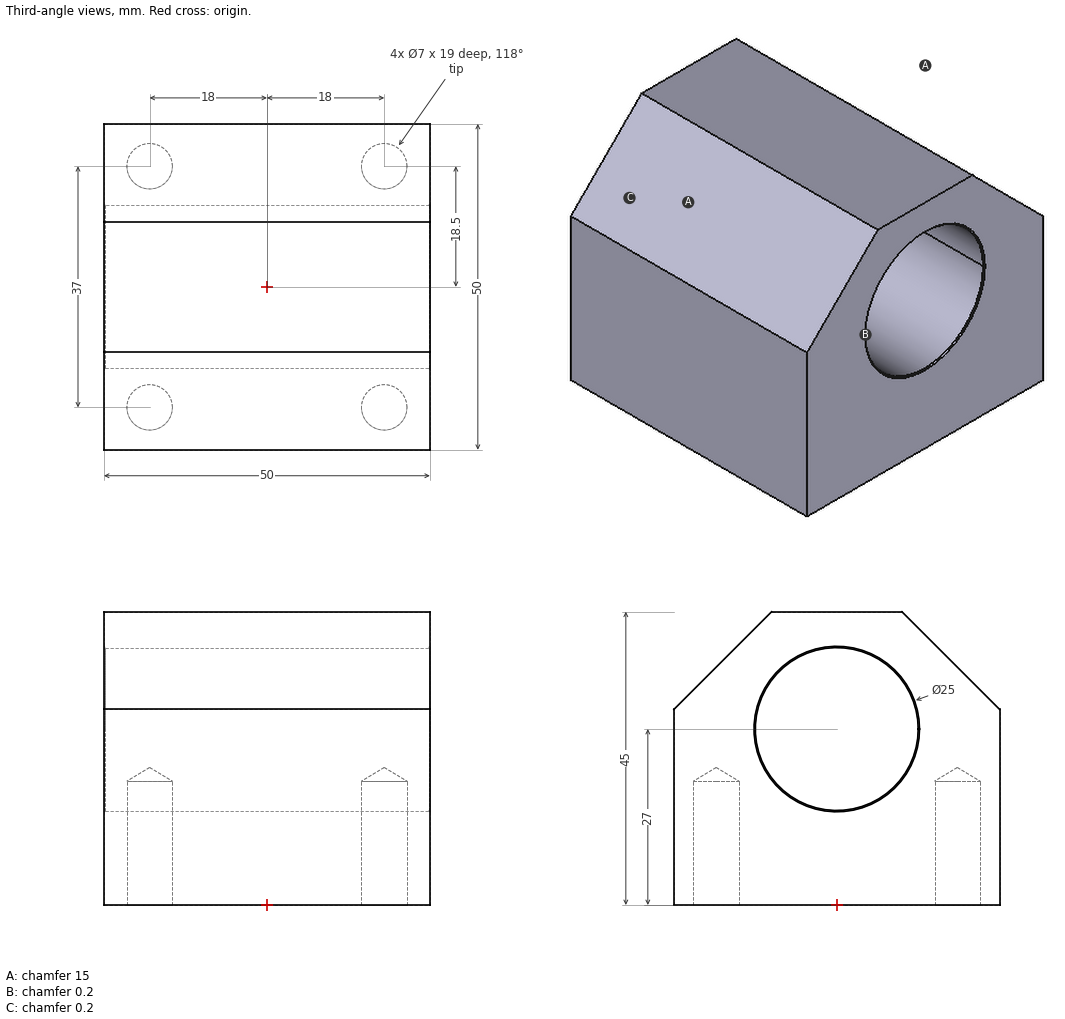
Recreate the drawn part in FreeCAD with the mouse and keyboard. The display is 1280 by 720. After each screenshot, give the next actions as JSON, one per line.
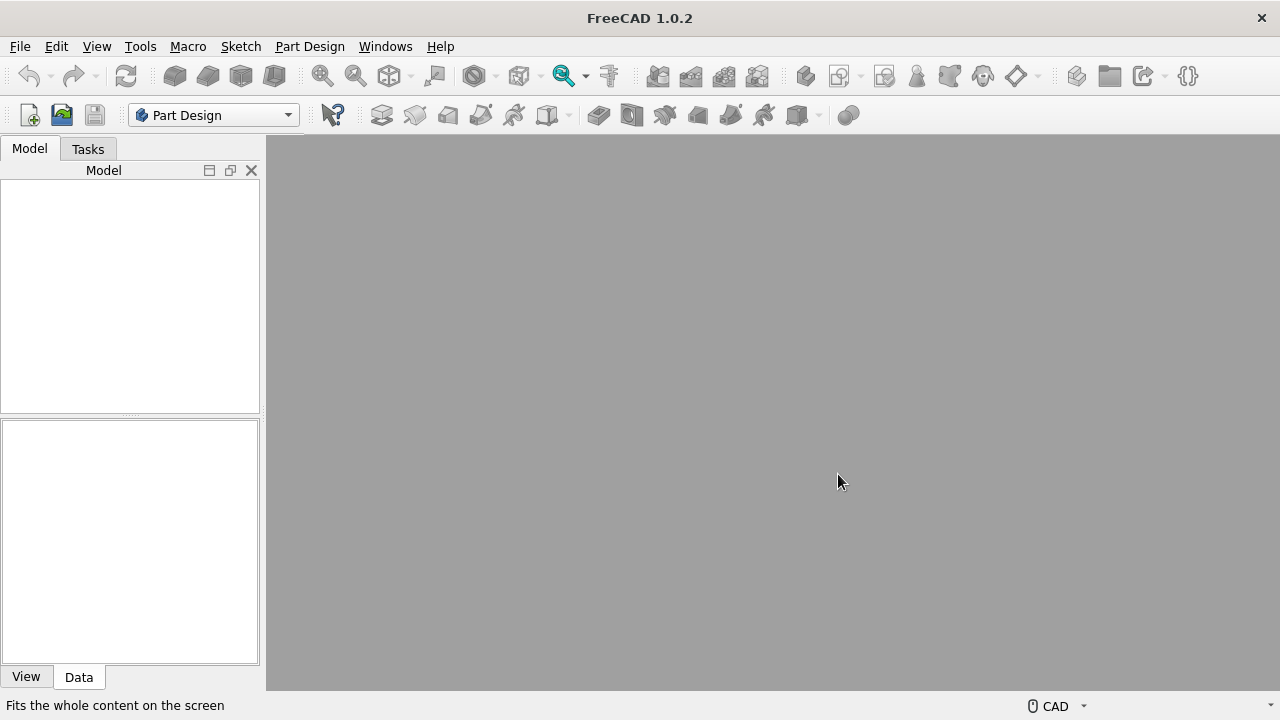
{"action": "left_click", "coordinate": [29, 116]}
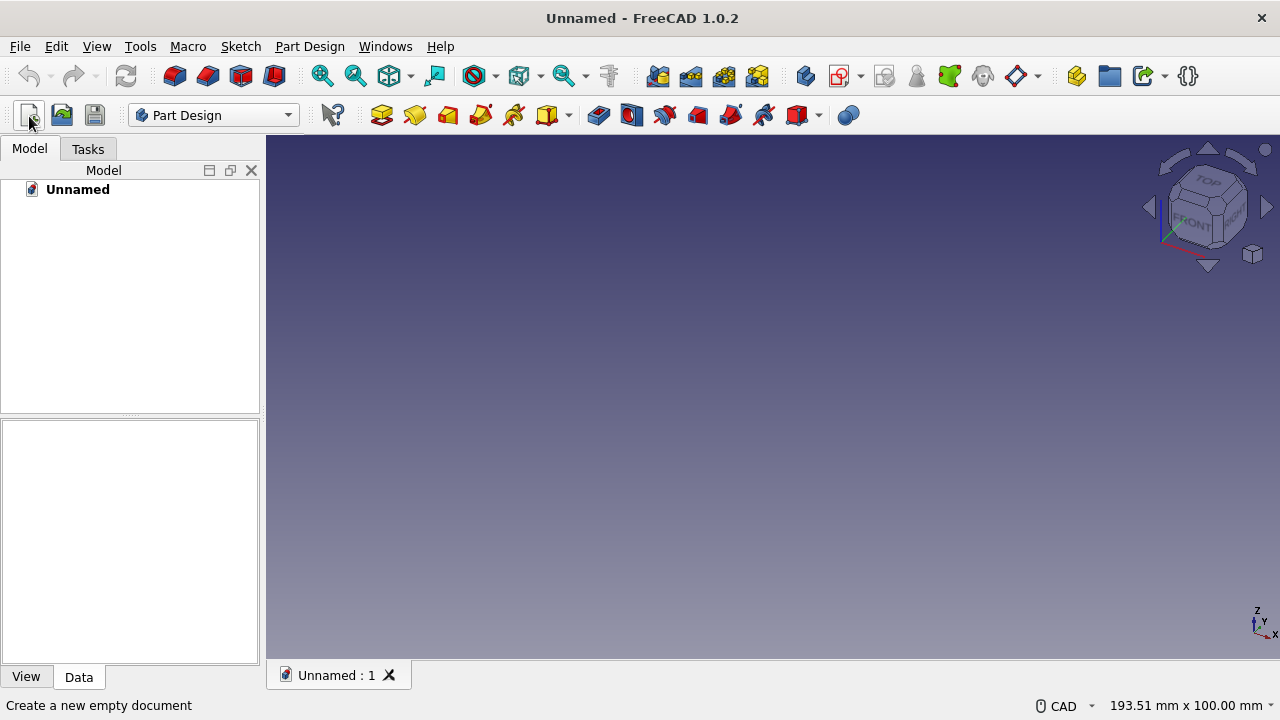
{"action": "left_click", "coordinate": [838, 76]}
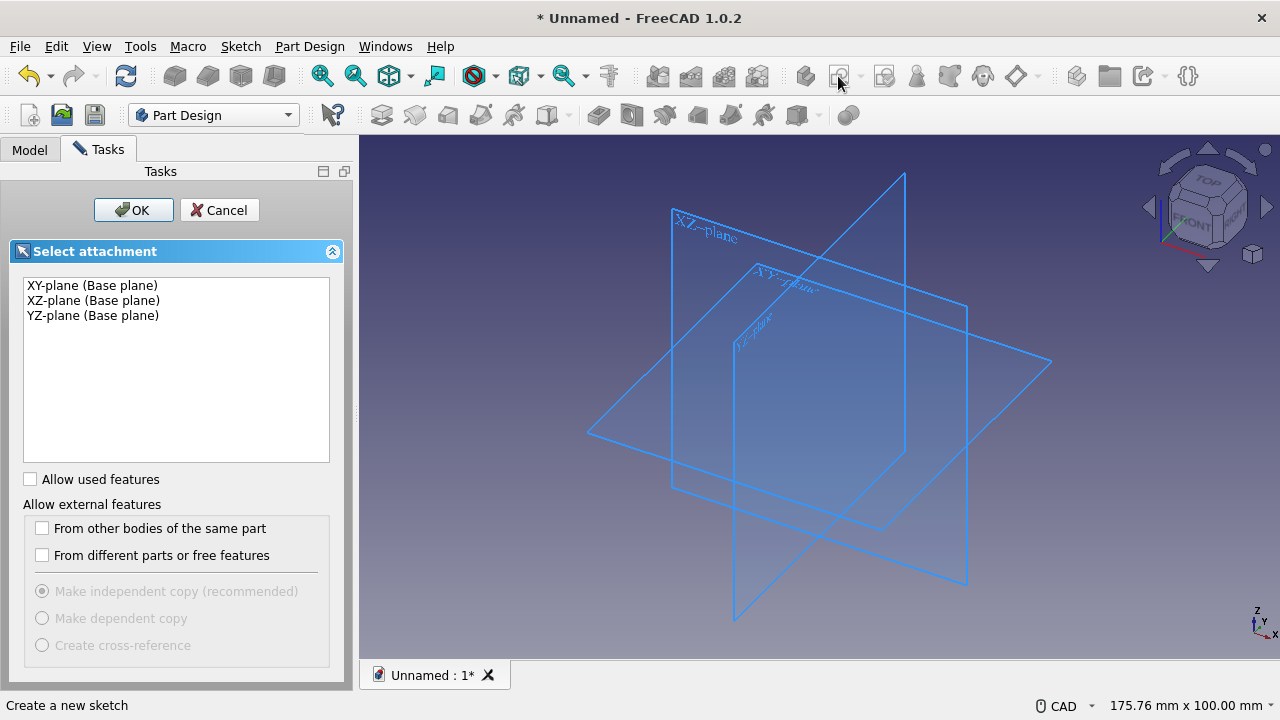
{"action": "left_click", "coordinate": [84, 286]}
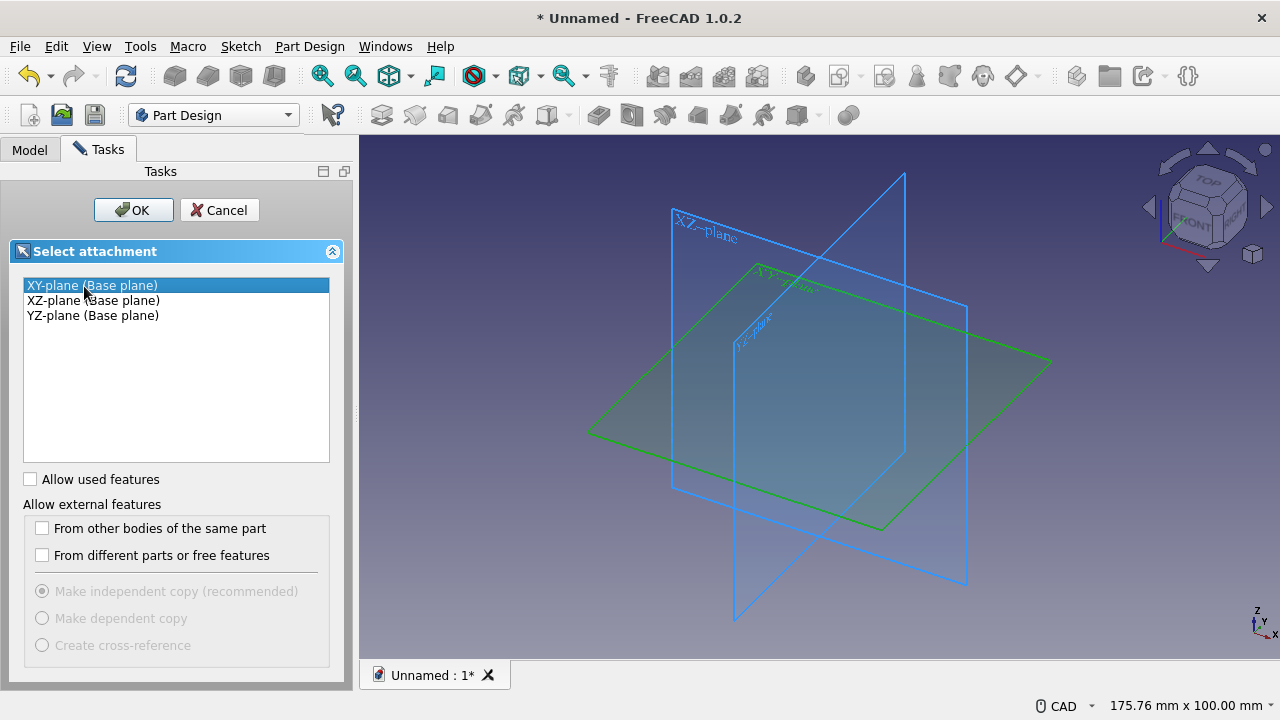
{"action": "left_click", "coordinate": [134, 210]}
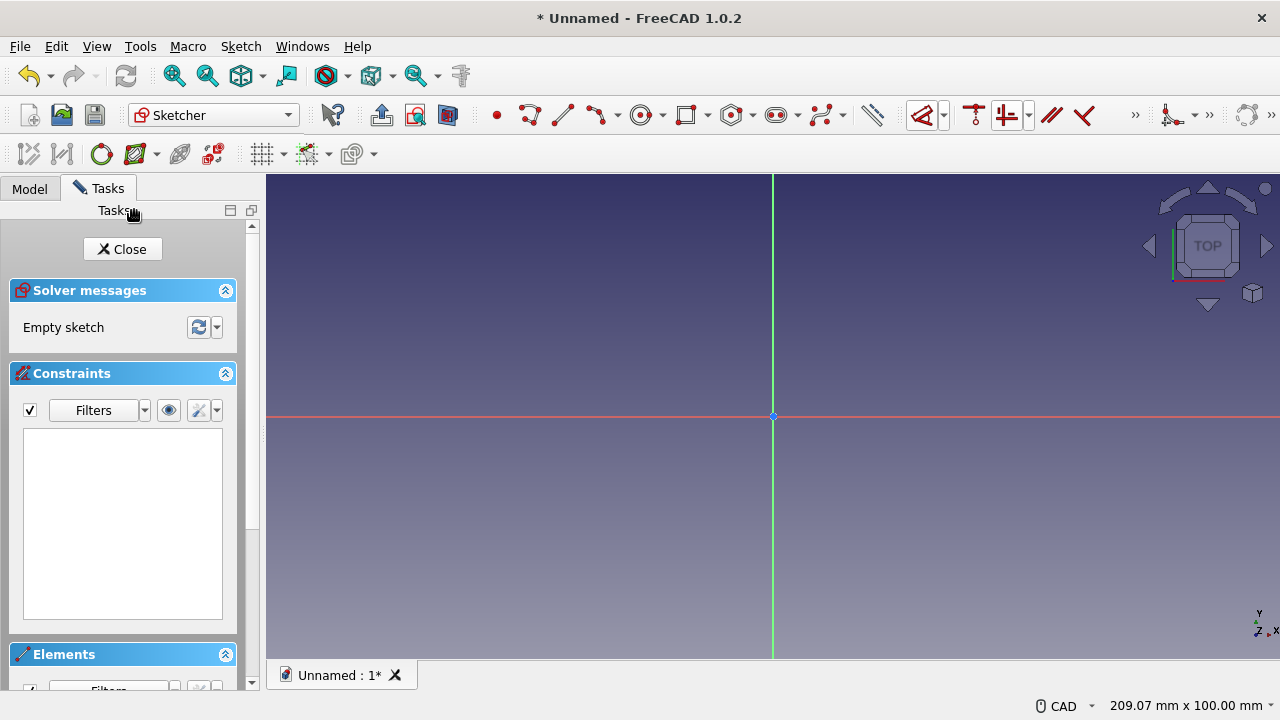
{"action": "left_click", "coordinate": [708, 116]}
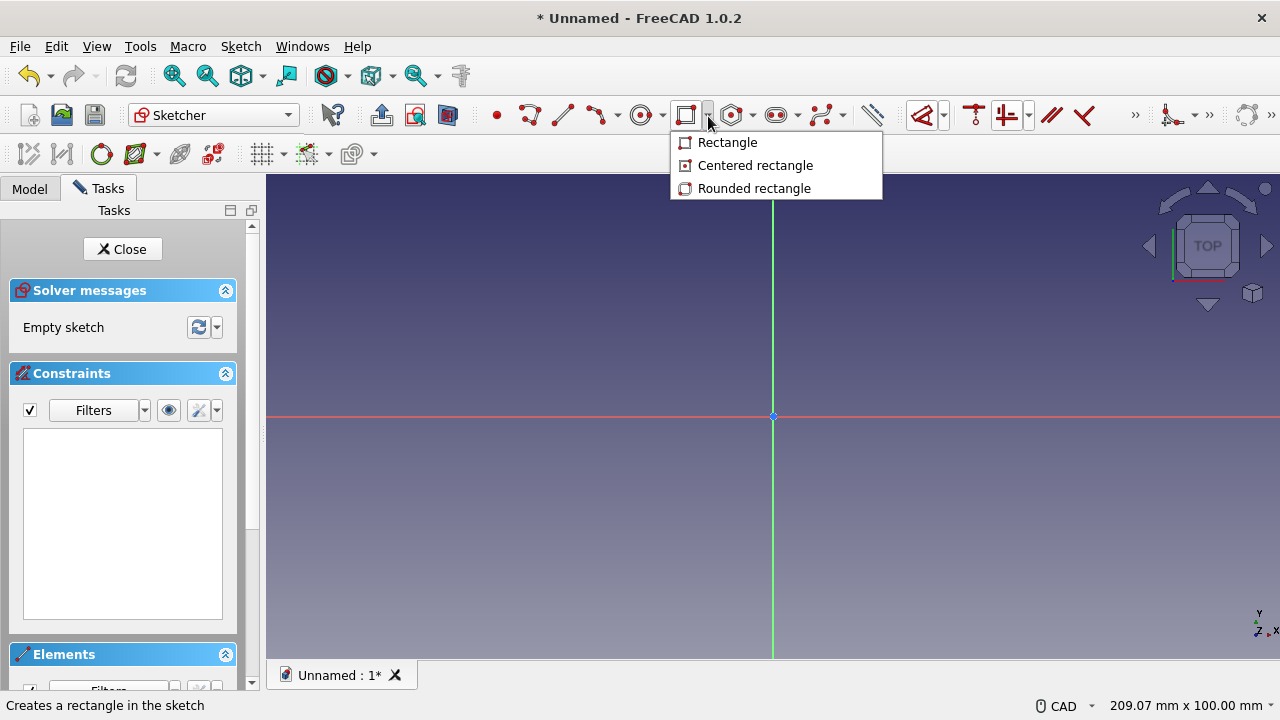
{"action": "left_click", "coordinate": [776, 166]}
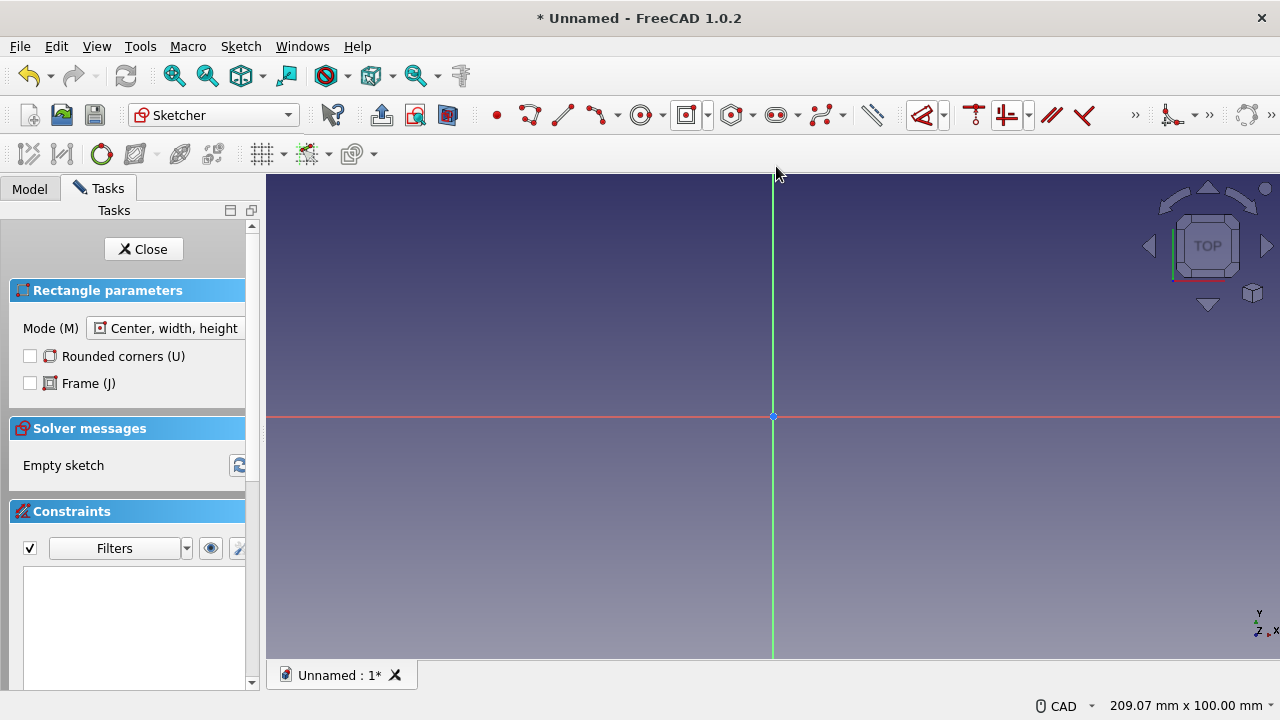
{"action": "left_click", "coordinate": [773, 416]}
{"action": "left_click", "coordinate": [894, 295]}
{"action": "key", "text": "Escape"}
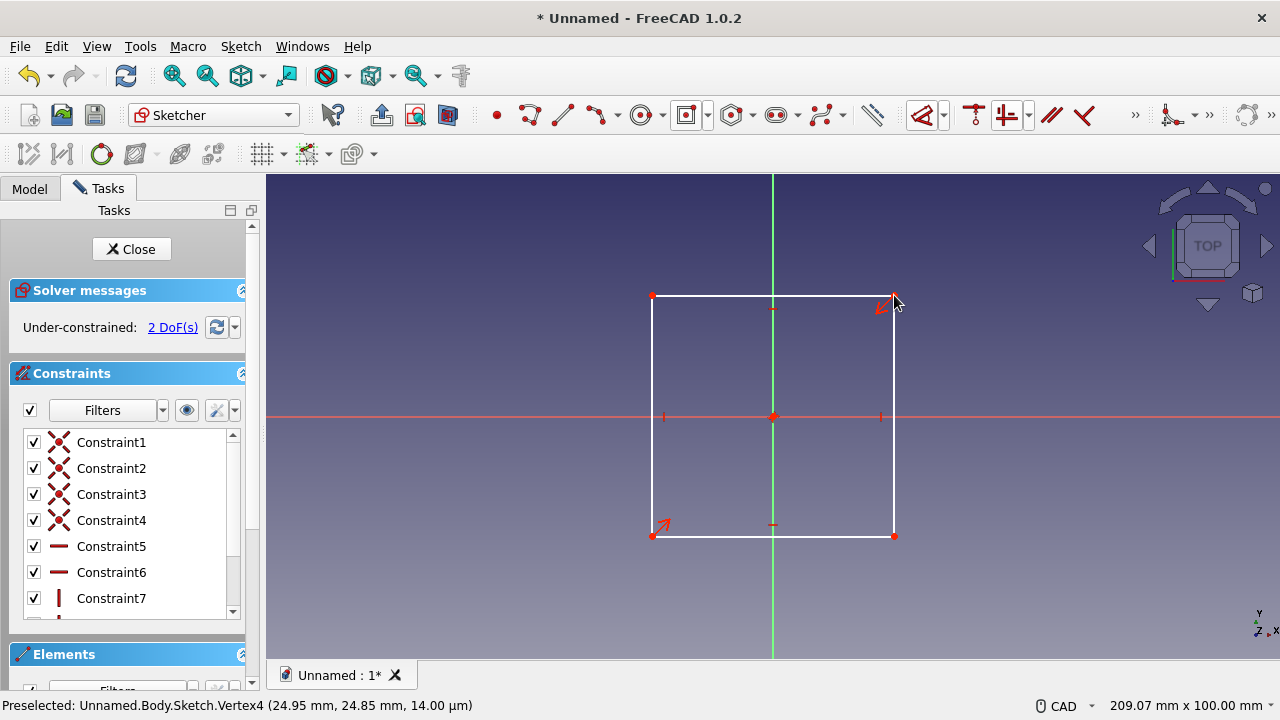
{"action": "left_click", "coordinate": [922, 116]}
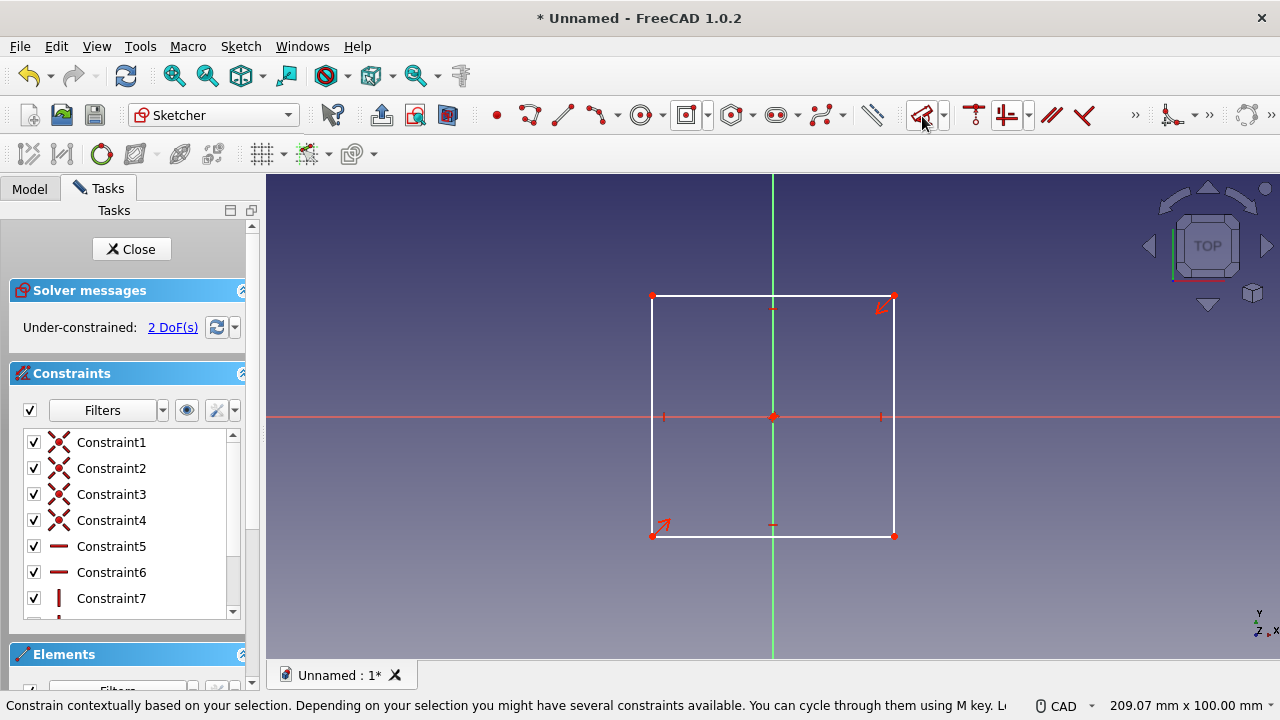
{"action": "left_click", "coordinate": [725, 537]}
{"action": "left_click", "coordinate": [717, 571]}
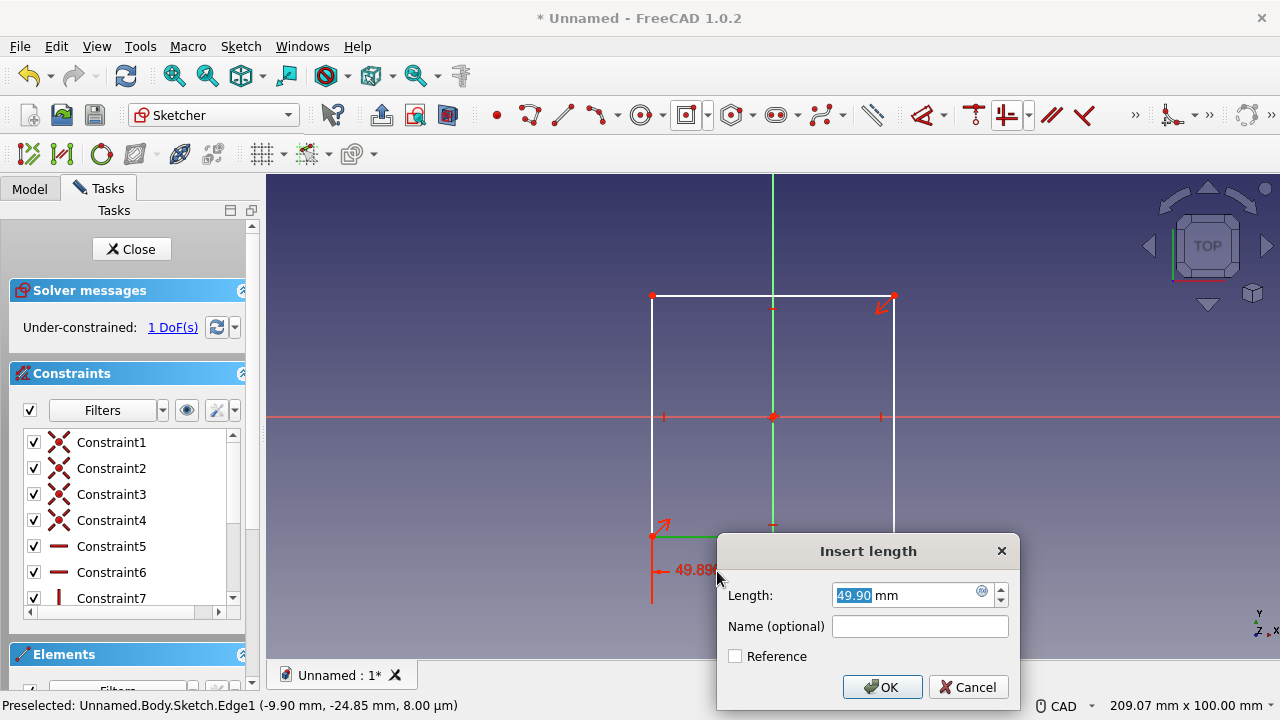
{"action": "type", "text": "50"}
{"action": "key", "text": "Return"}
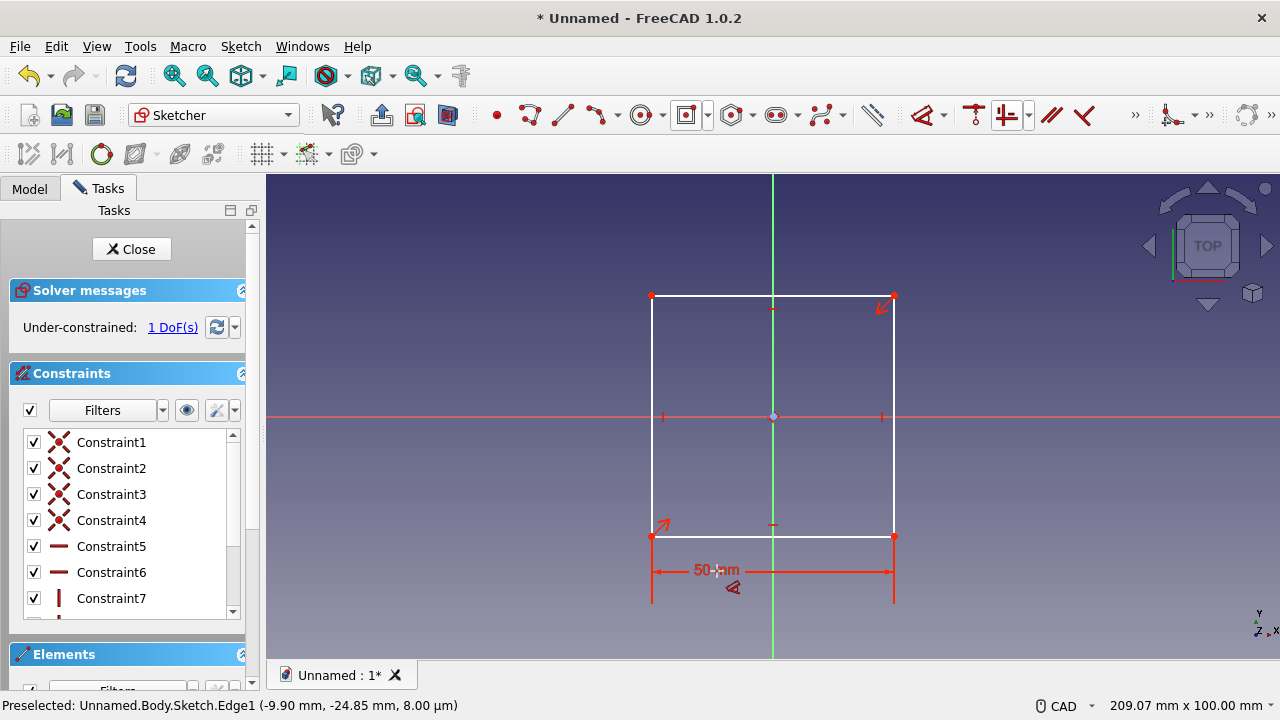
{"action": "left_click", "coordinate": [894, 465]}
{"action": "left_click", "coordinate": [928, 361]}